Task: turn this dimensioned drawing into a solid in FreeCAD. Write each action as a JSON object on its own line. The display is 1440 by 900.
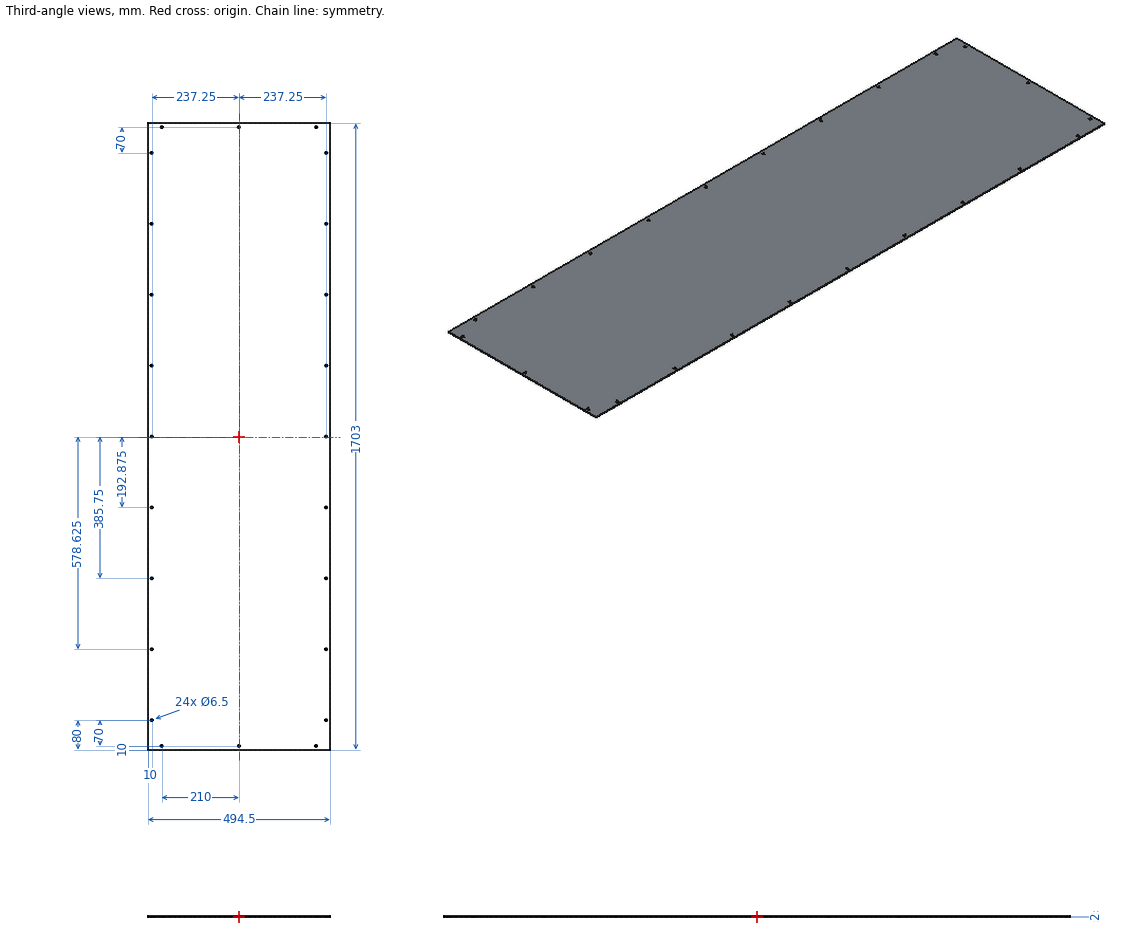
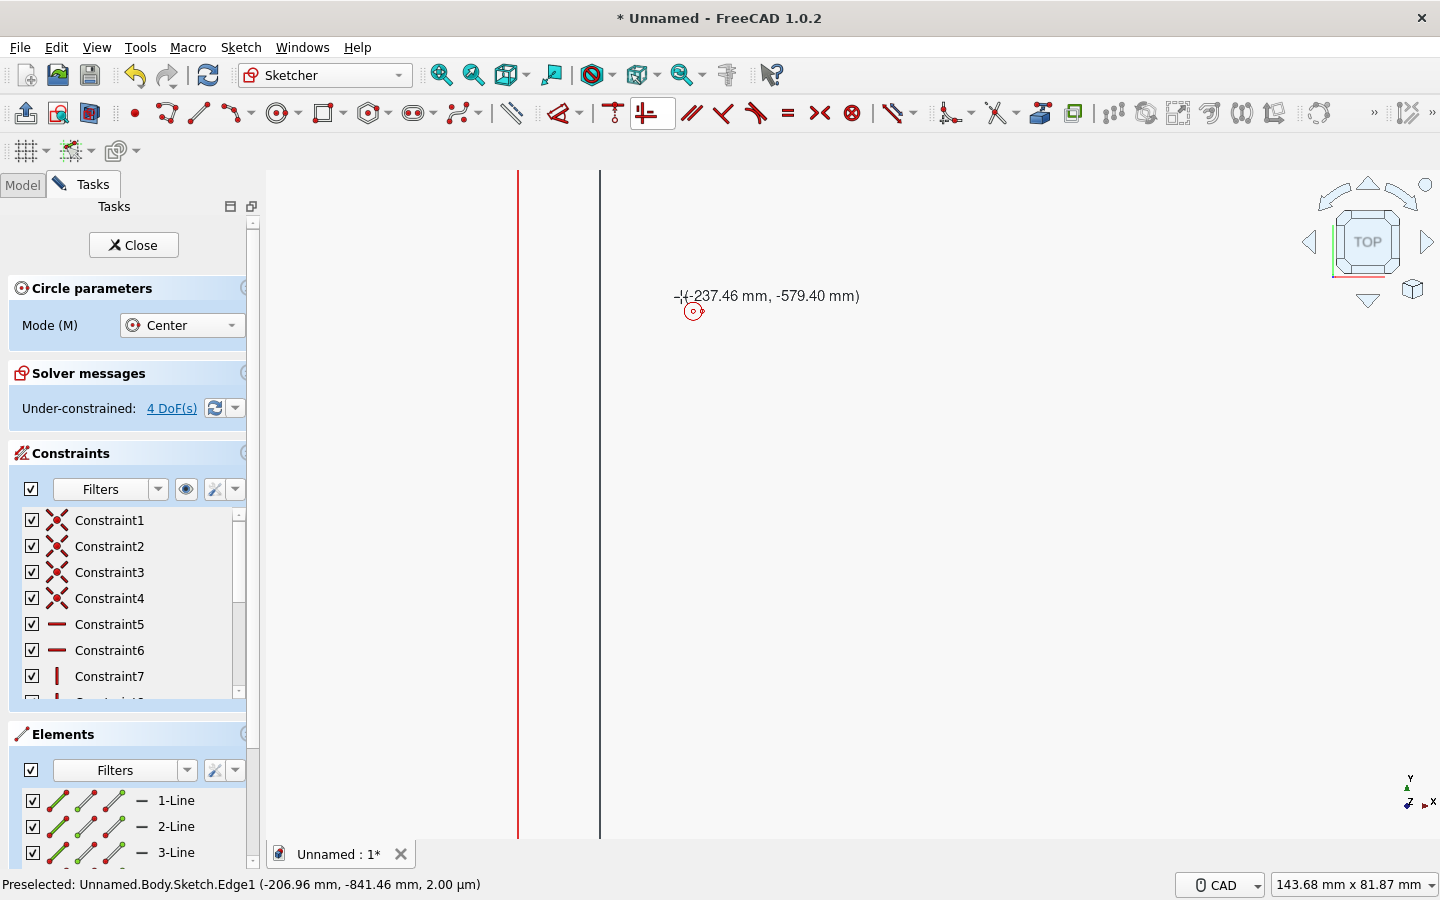
{"action": "scroll", "coordinate": [721, 675], "scroll_direction": "down", "scroll_amount": 17}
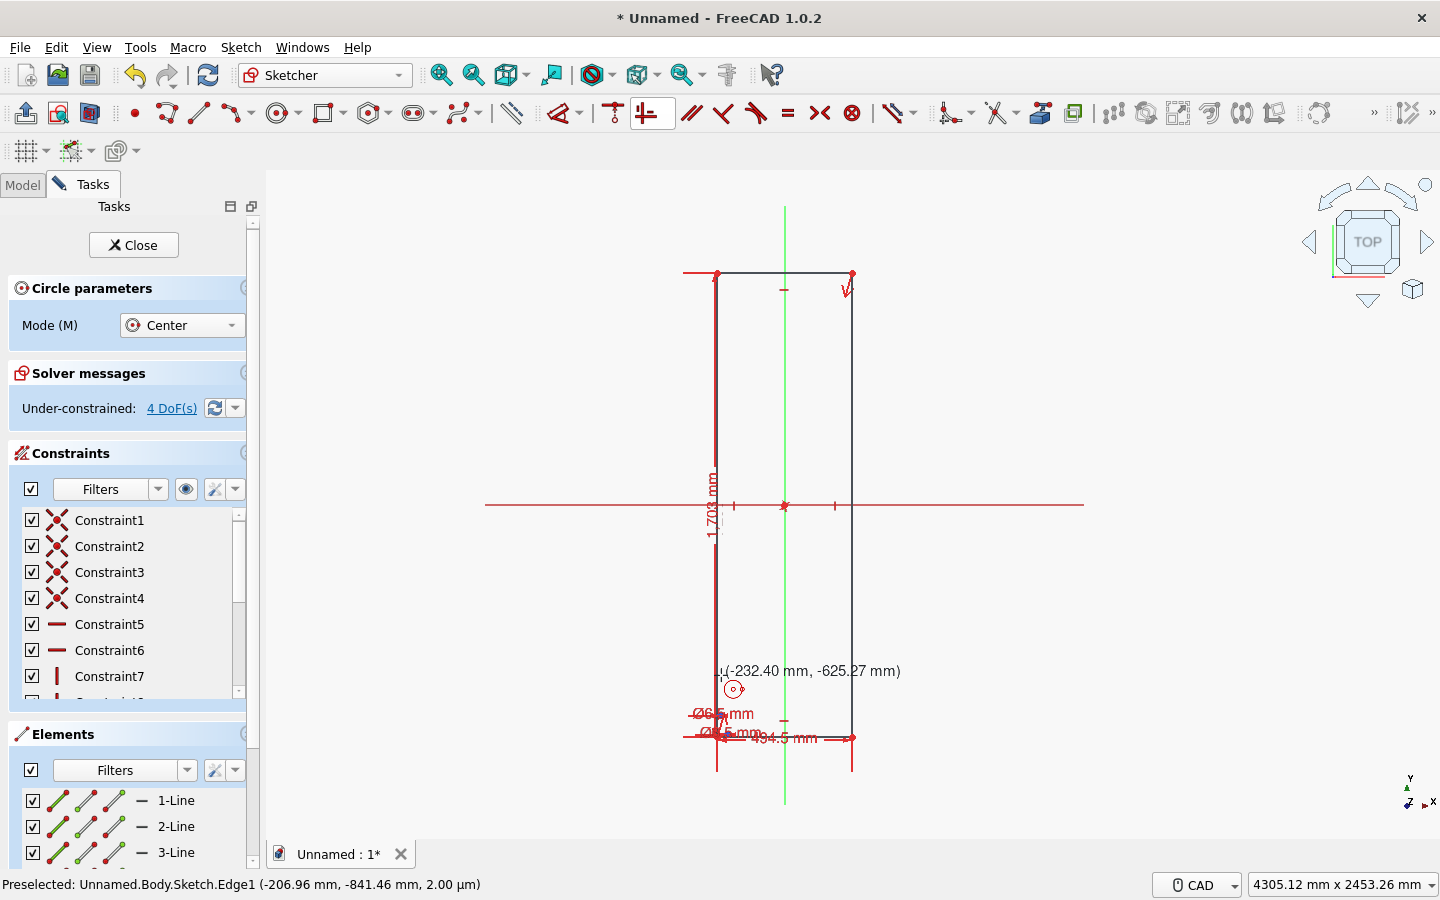
{"action": "scroll", "coordinate": [720, 663], "scroll_direction": "up", "scroll_amount": 9}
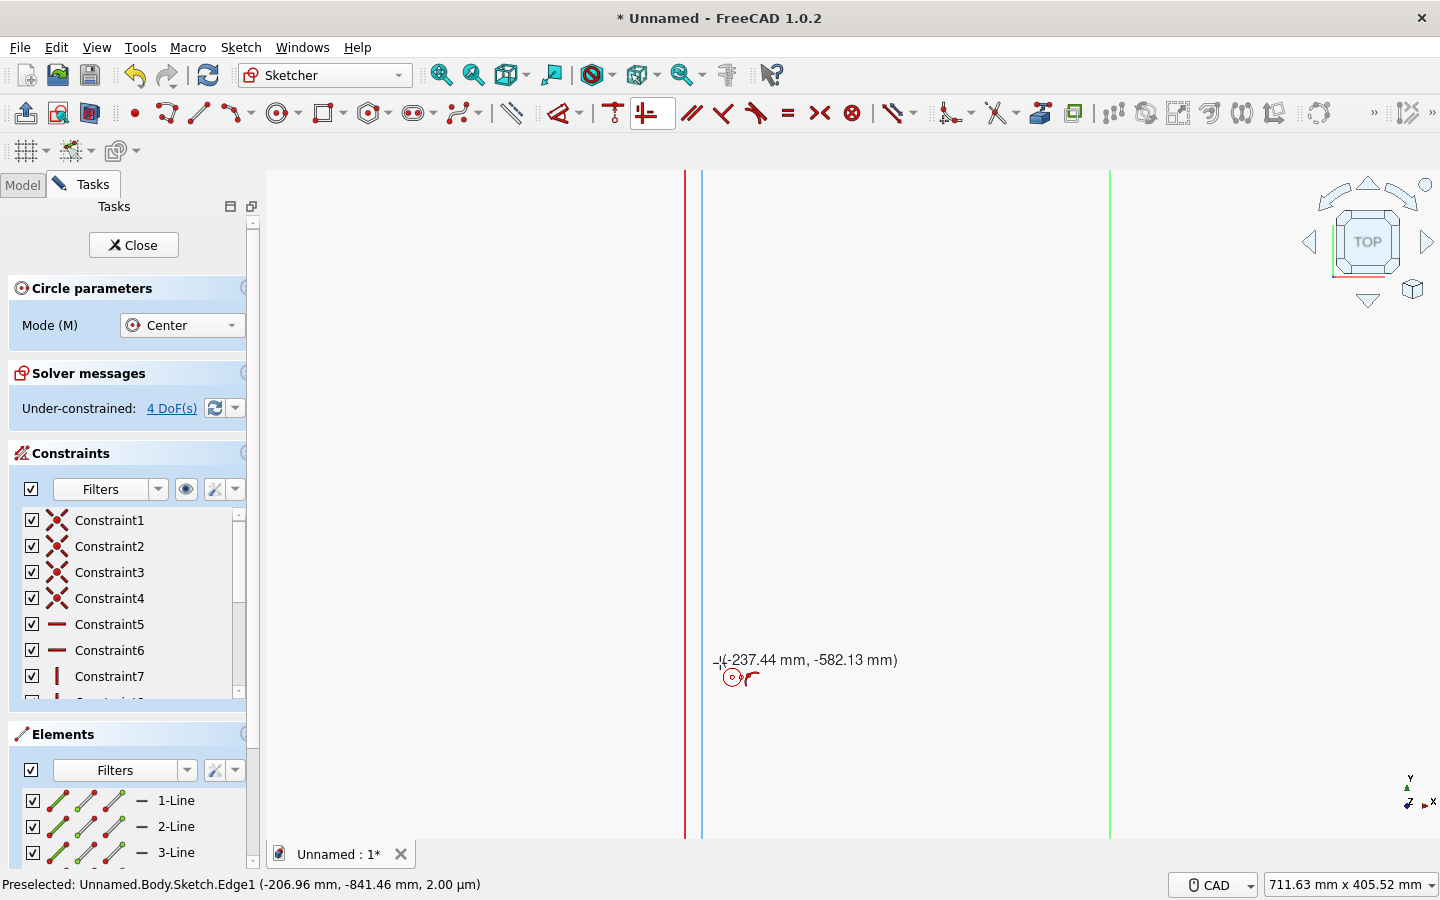
{"action": "left_click", "coordinate": [718, 660]}
{"action": "mouse_move", "coordinate": [722, 656]}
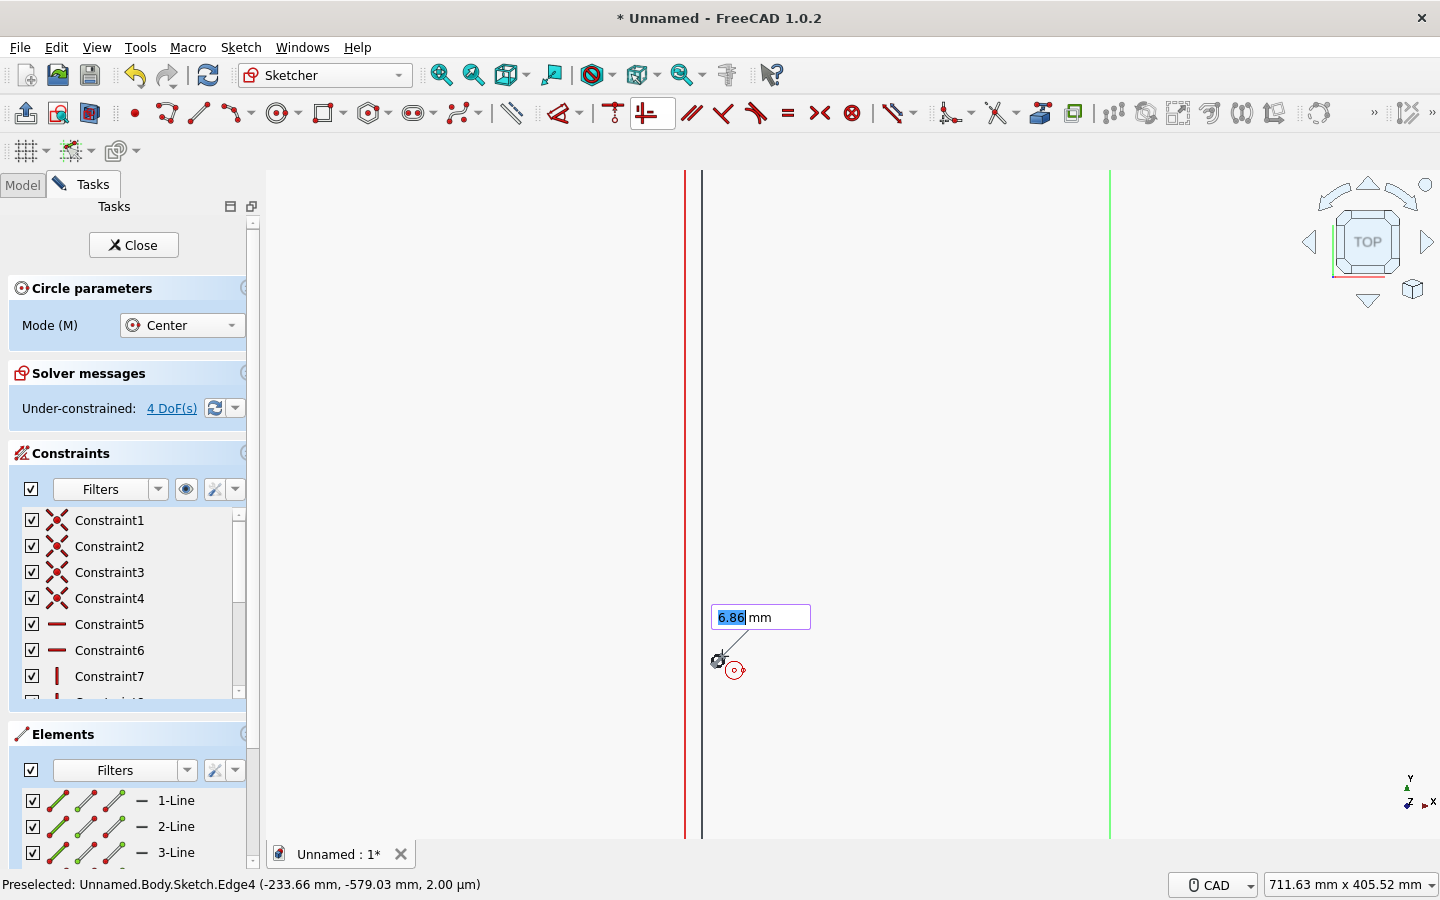
{"action": "type", "text": "6.5"}
{"action": "key", "text": "Return"}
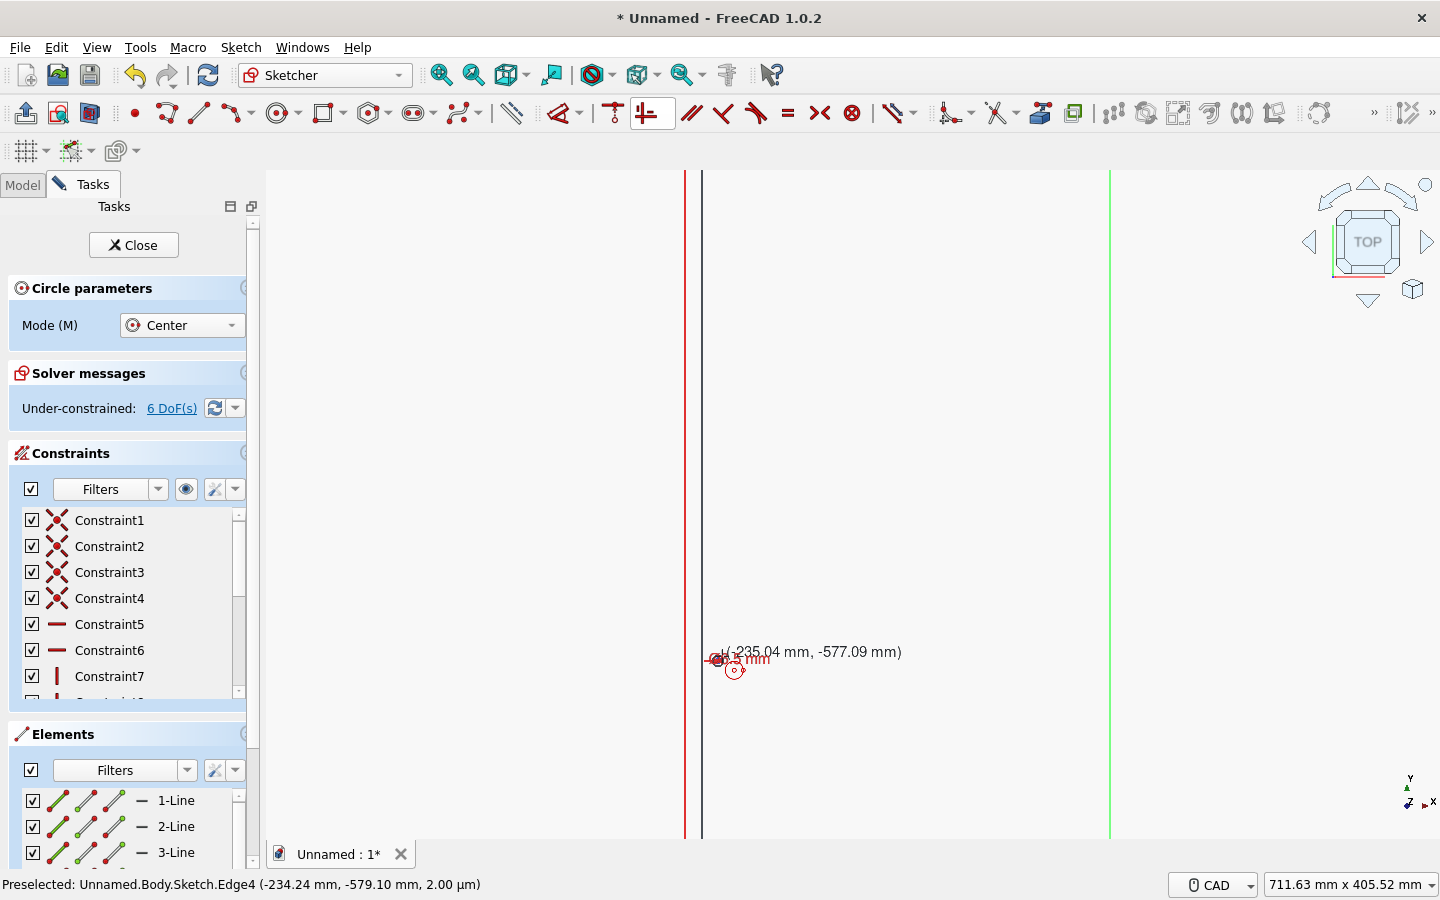
{"action": "scroll", "coordinate": [718, 341], "scroll_direction": "up", "scroll_amount": 8}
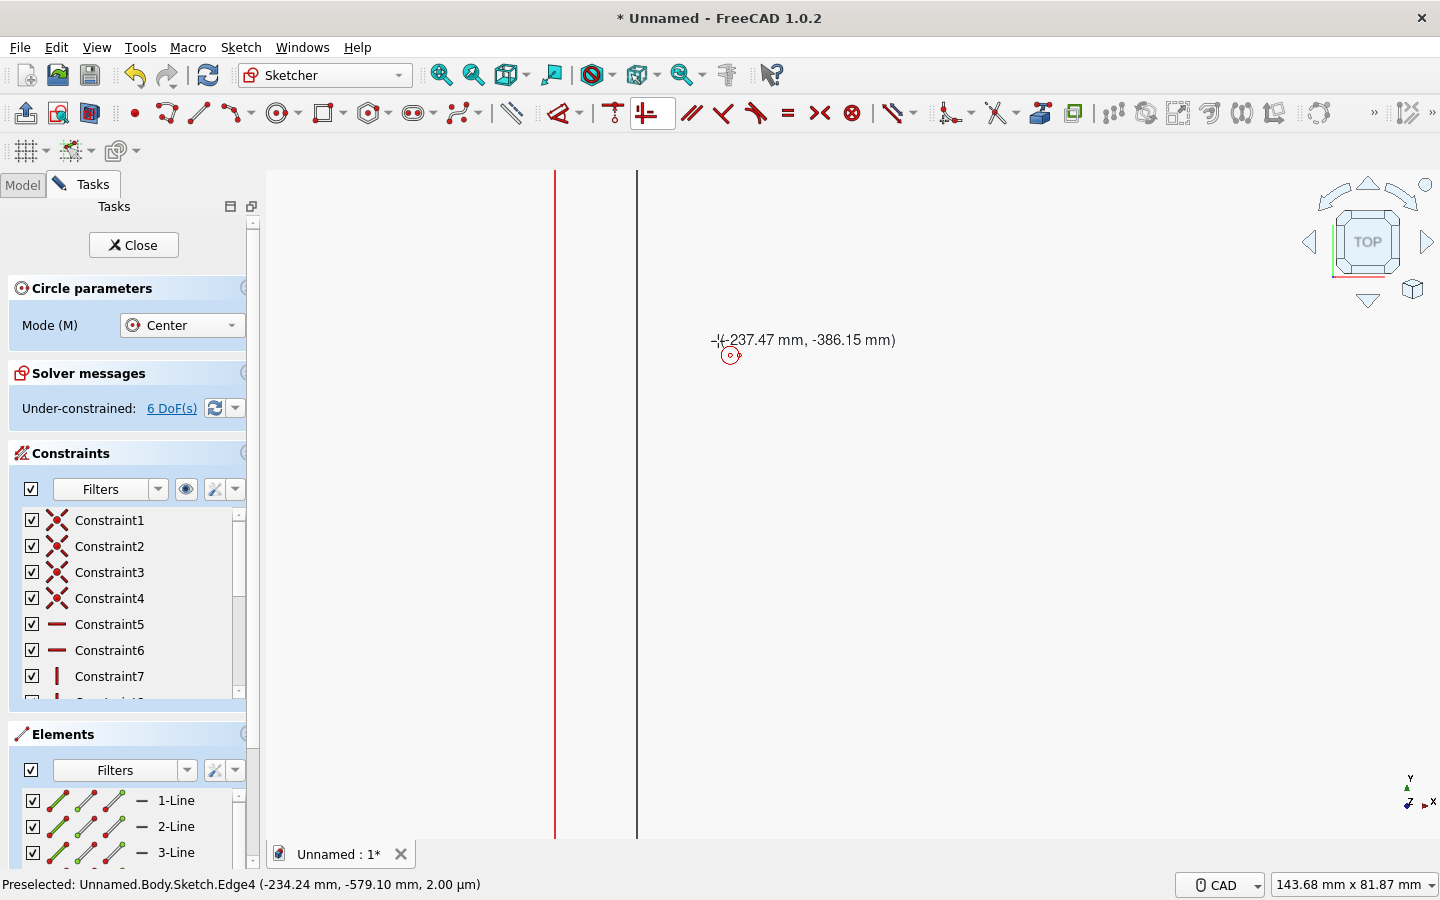
{"action": "scroll", "coordinate": [720, 619], "scroll_direction": "down", "scroll_amount": 17}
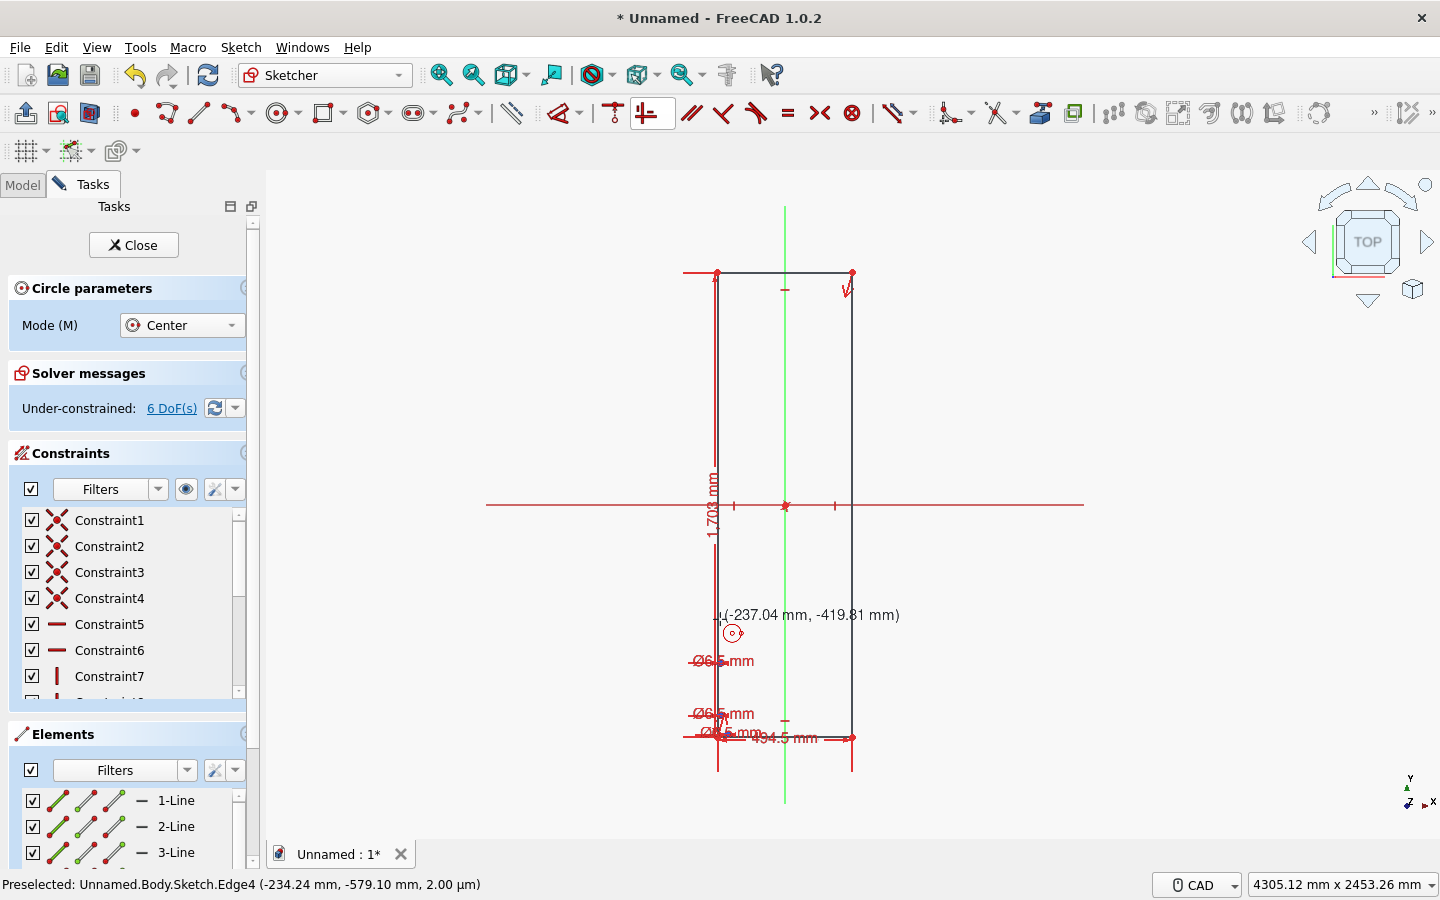
{"action": "scroll", "coordinate": [720, 610], "scroll_direction": "up", "scroll_amount": 9}